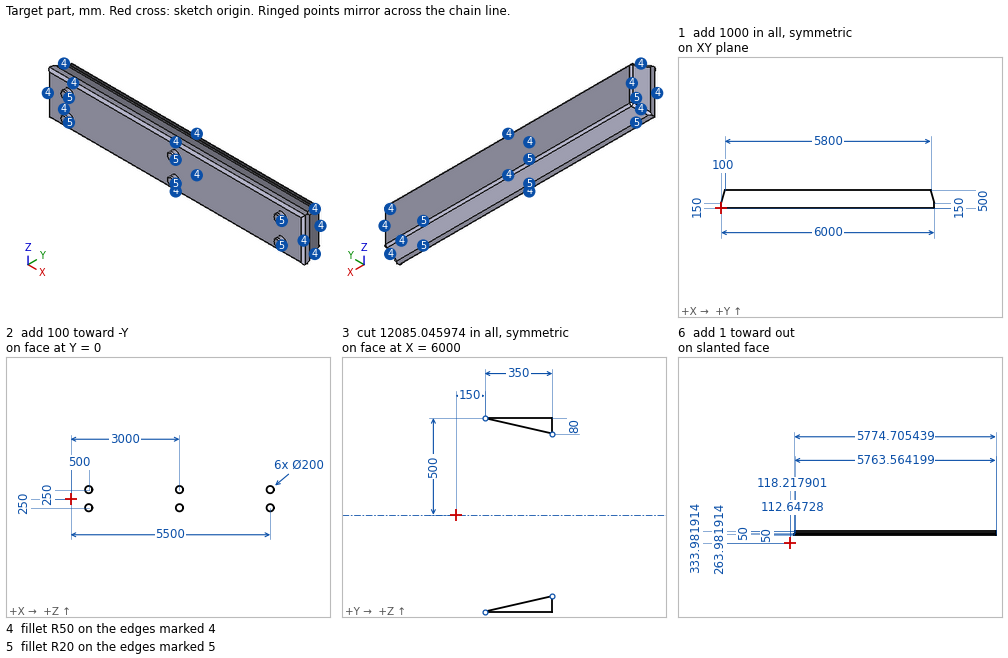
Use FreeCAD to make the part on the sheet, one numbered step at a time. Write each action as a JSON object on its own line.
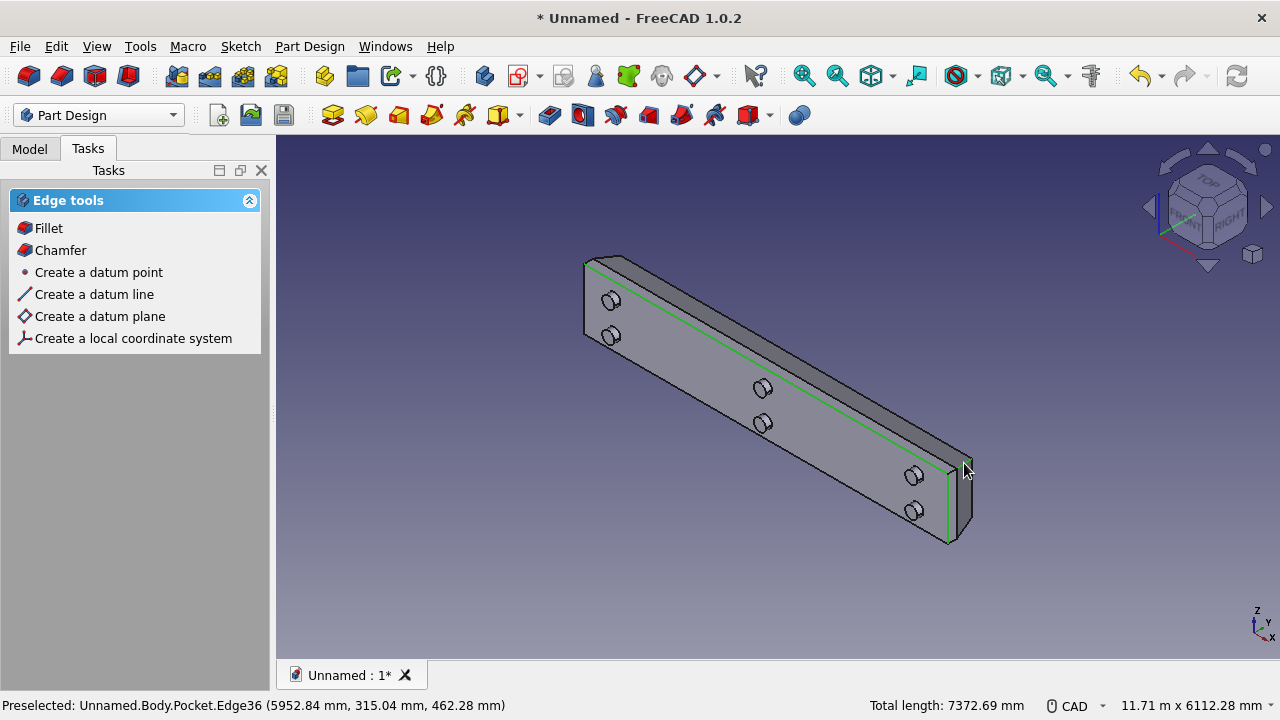
{"action": "key", "text": "1"}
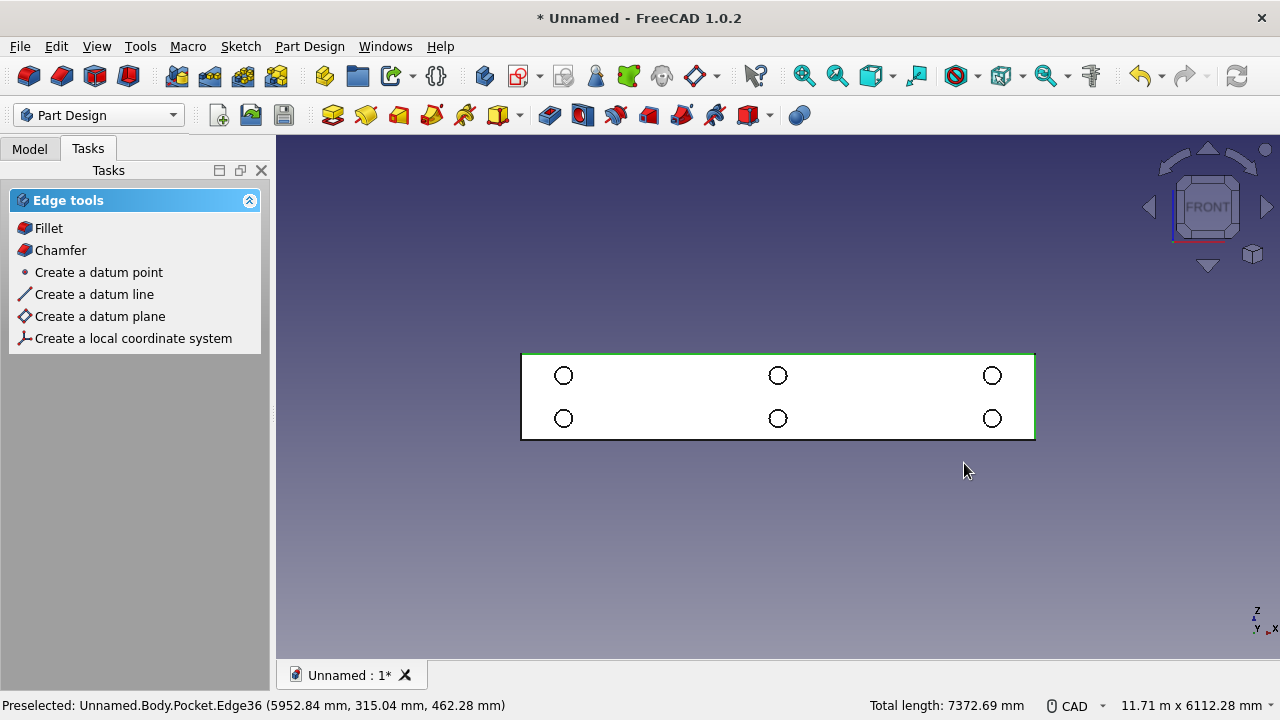
{"action": "left_click", "coordinate": [778, 439], "text": "ctrl"}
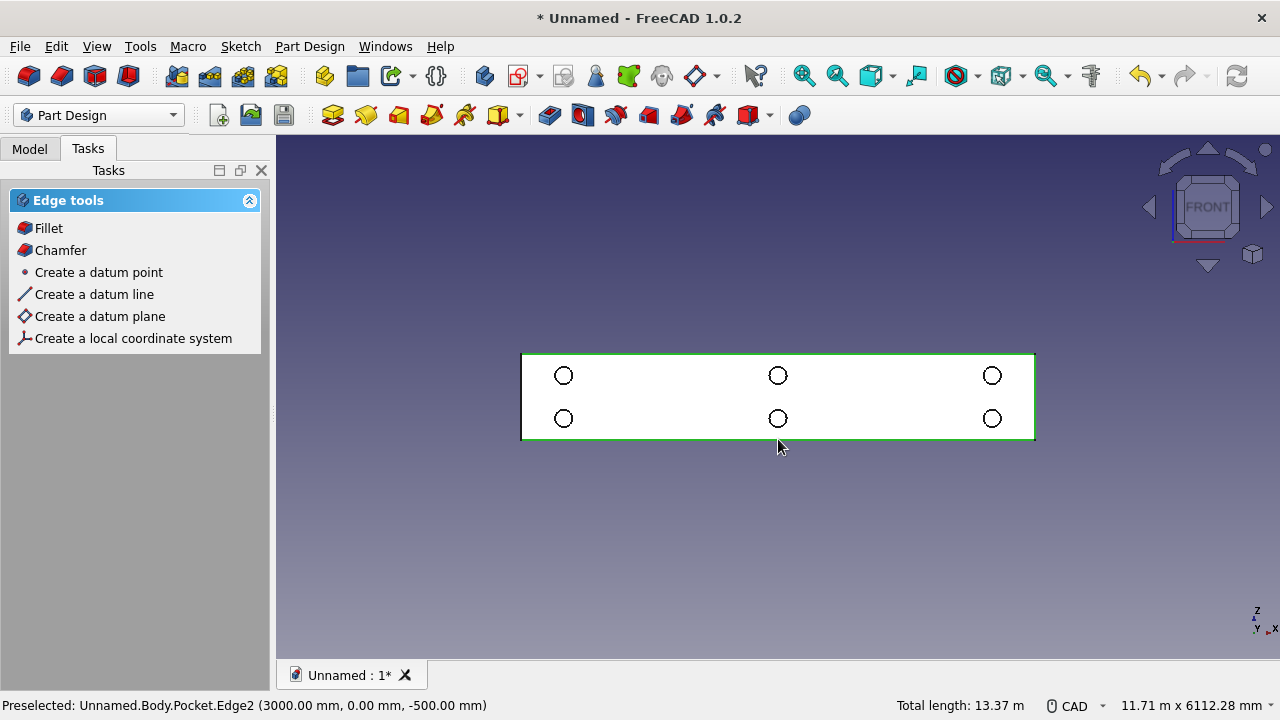
{"action": "left_click", "coordinate": [521, 396], "text": "ctrl"}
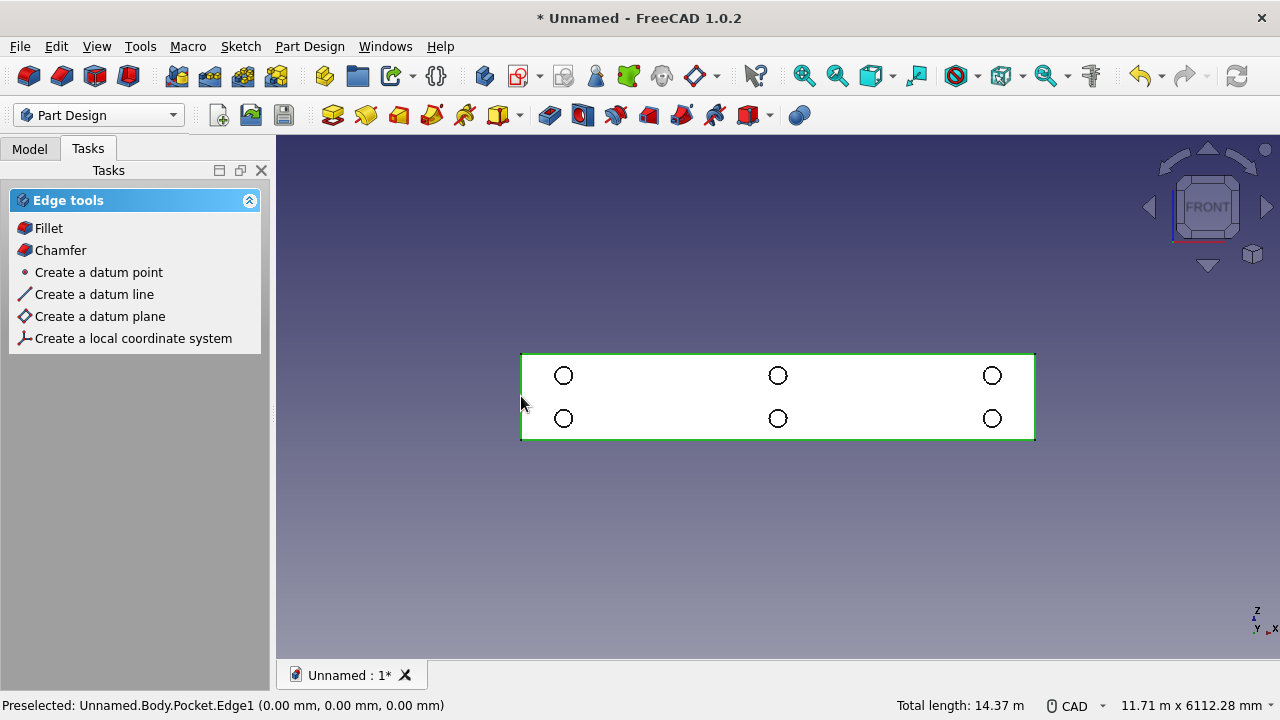
{"action": "key", "text": "3"}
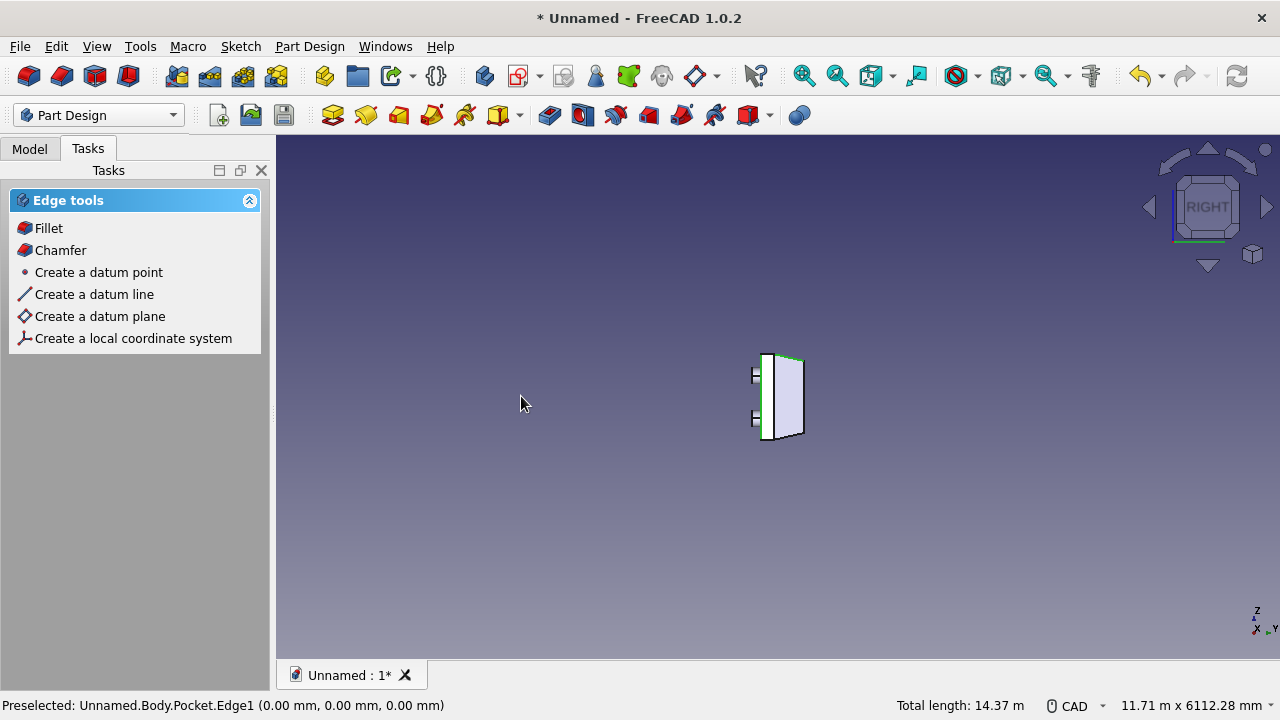
{"action": "key", "text": "v f"}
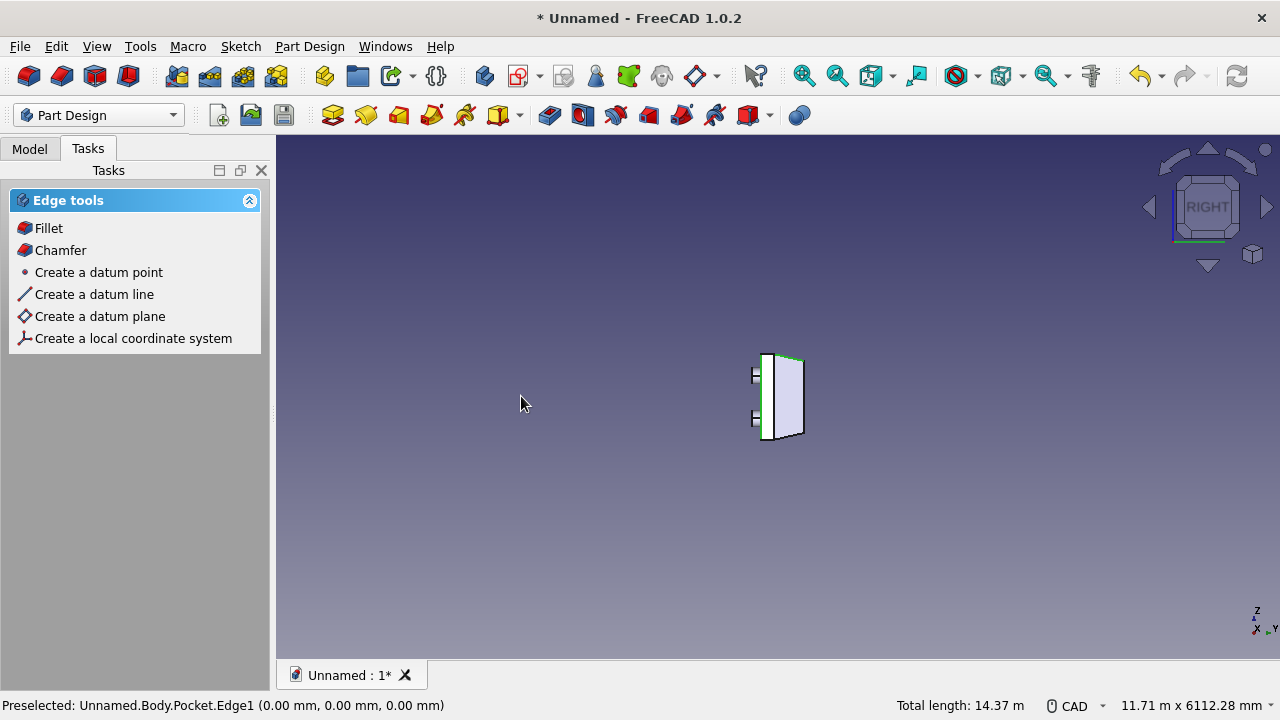
{"action": "key", "text": "5"}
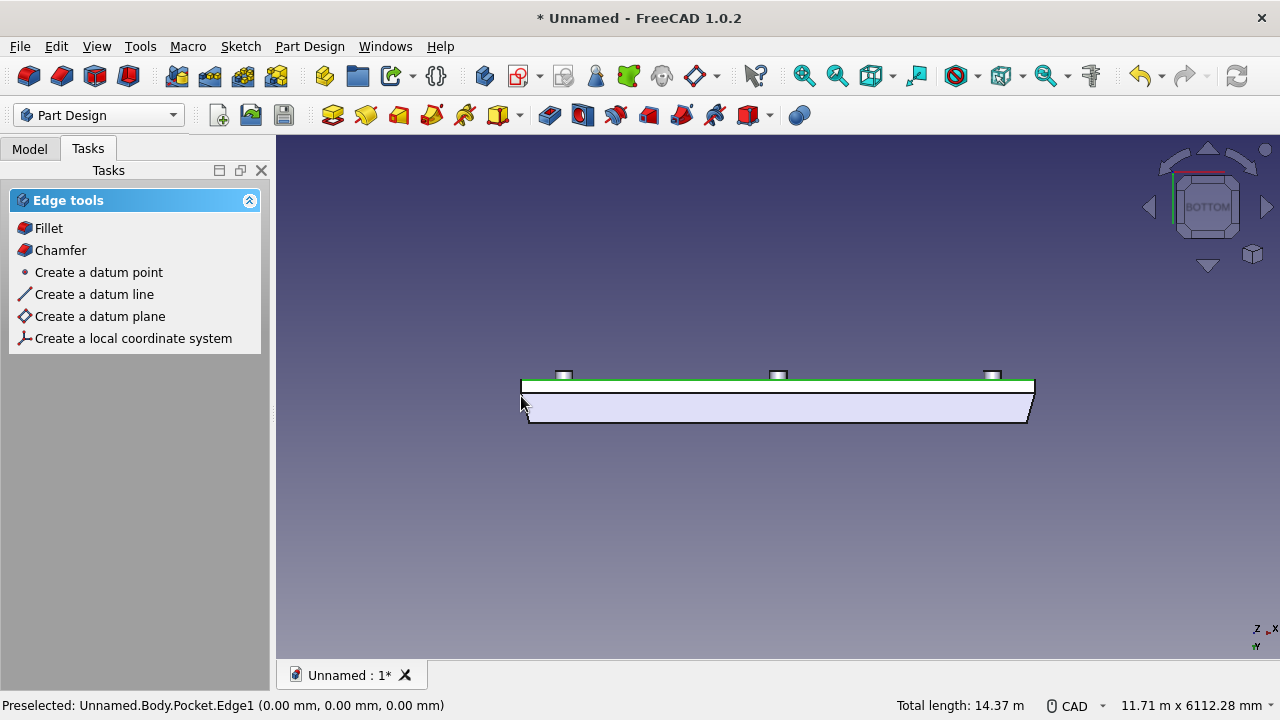
{"action": "key", "text": "4"}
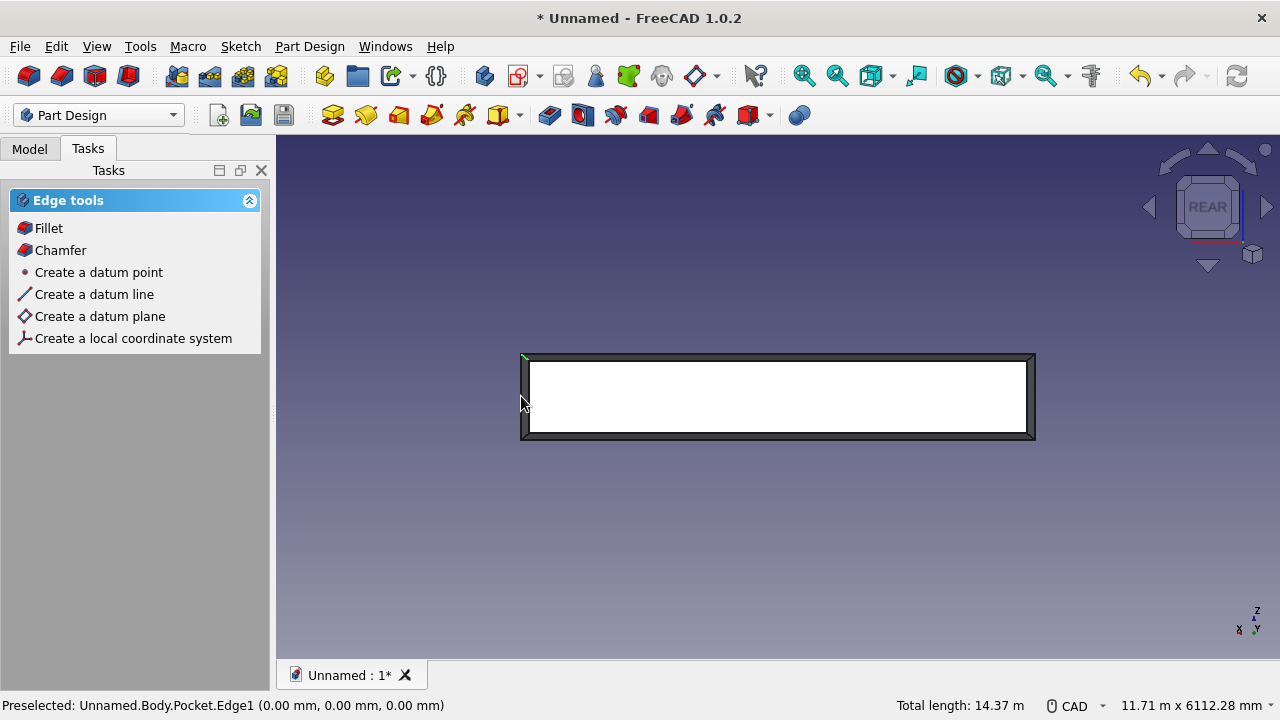
{"action": "left_click", "coordinate": [636, 396], "text": "ctrl"}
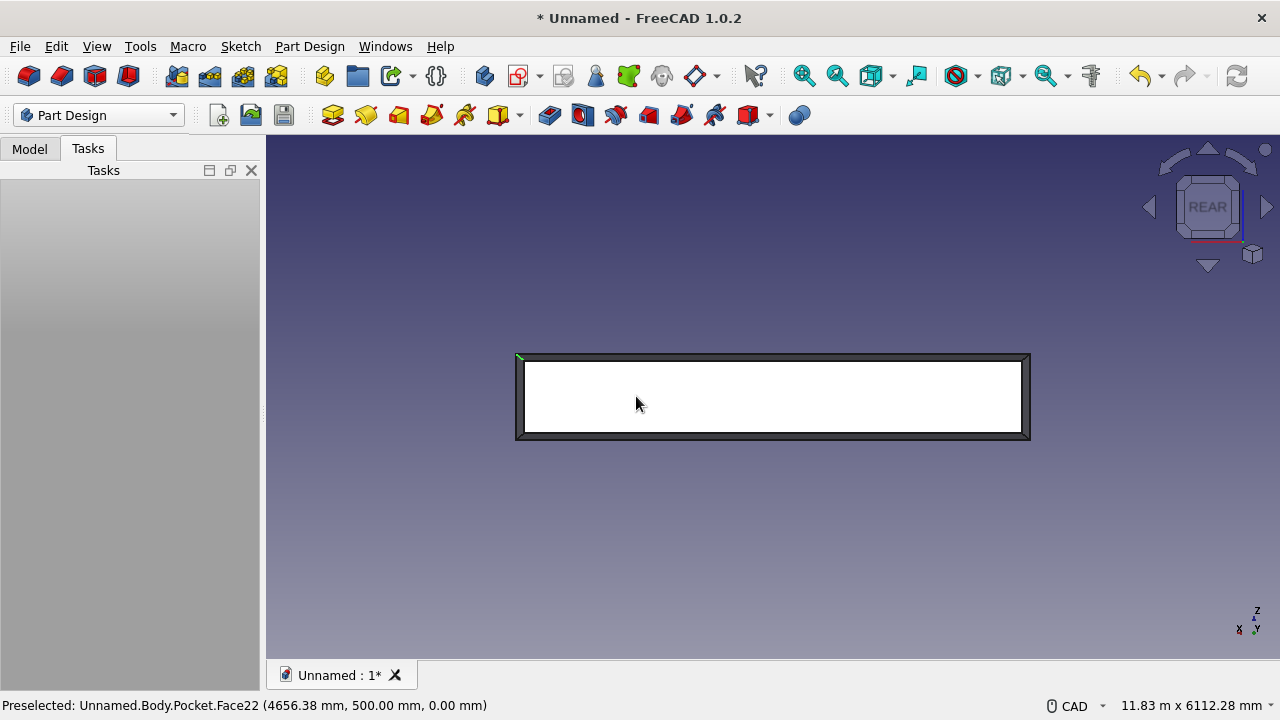
{"action": "left_click", "coordinate": [519, 436], "text": "ctrl"}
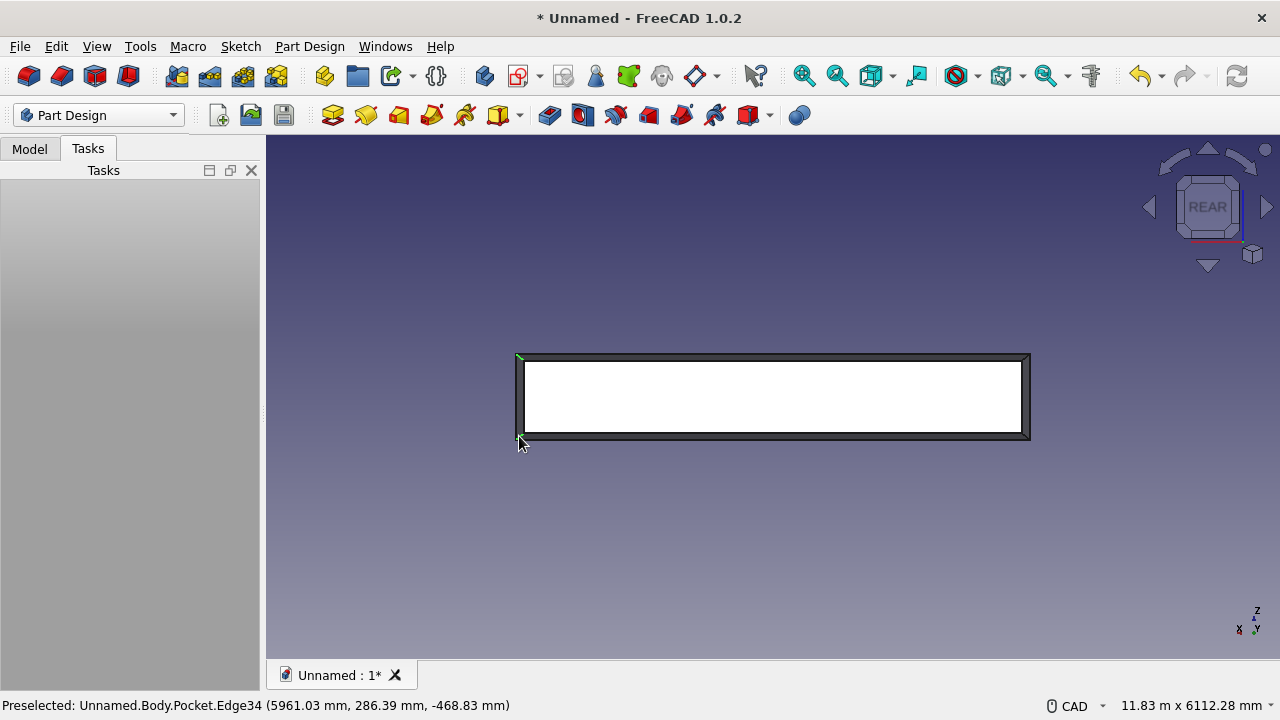
{"action": "left_click", "coordinate": [1027, 356], "text": "ctrl"}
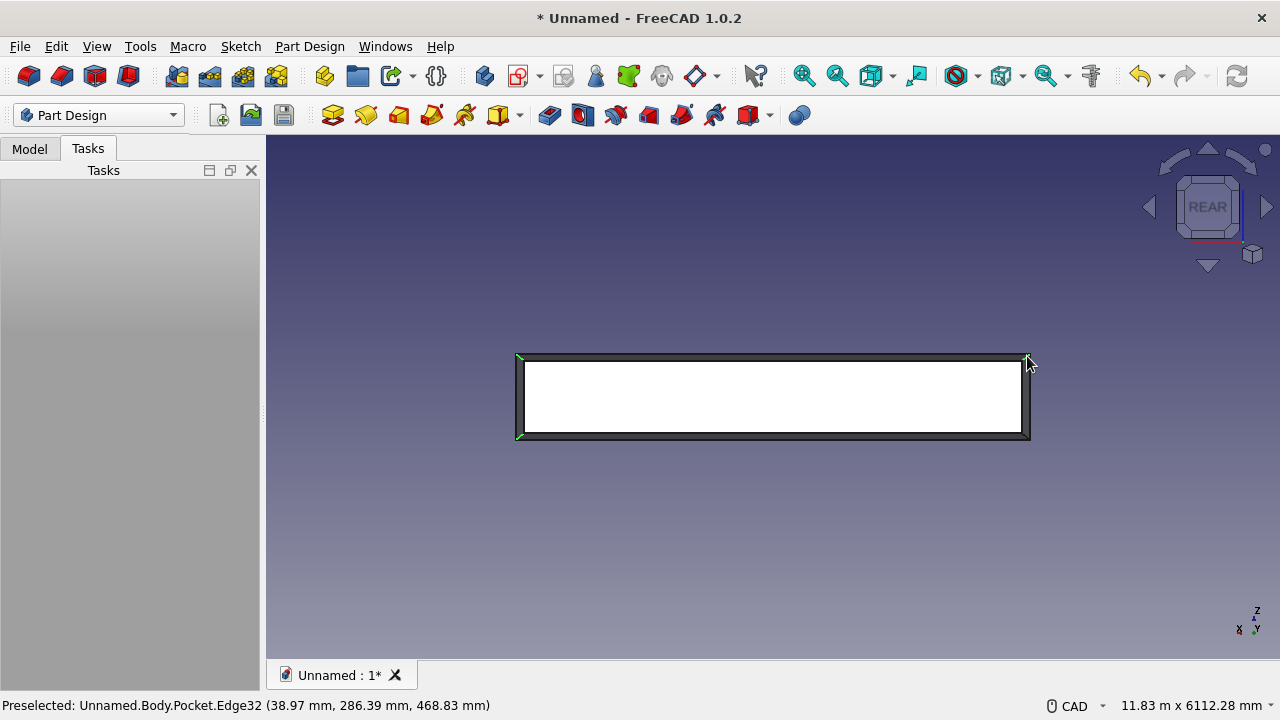
{"action": "left_click", "coordinate": [1027, 436], "text": "ctrl"}